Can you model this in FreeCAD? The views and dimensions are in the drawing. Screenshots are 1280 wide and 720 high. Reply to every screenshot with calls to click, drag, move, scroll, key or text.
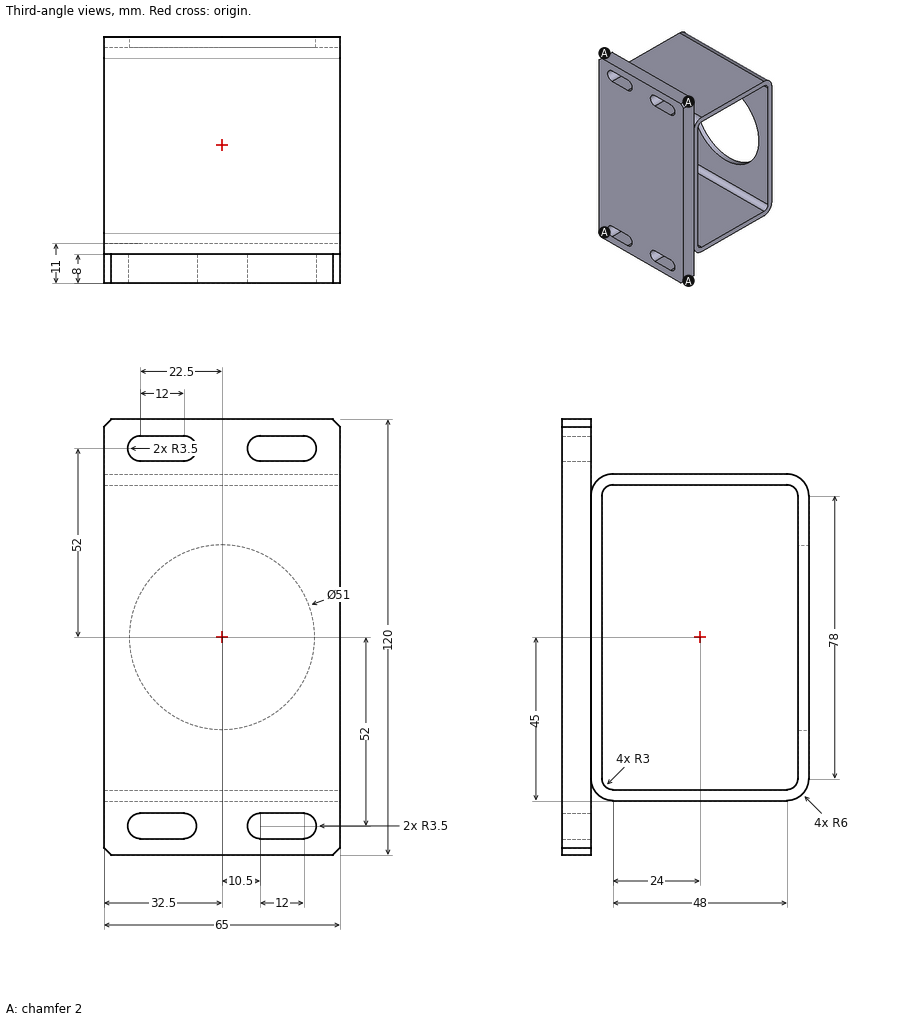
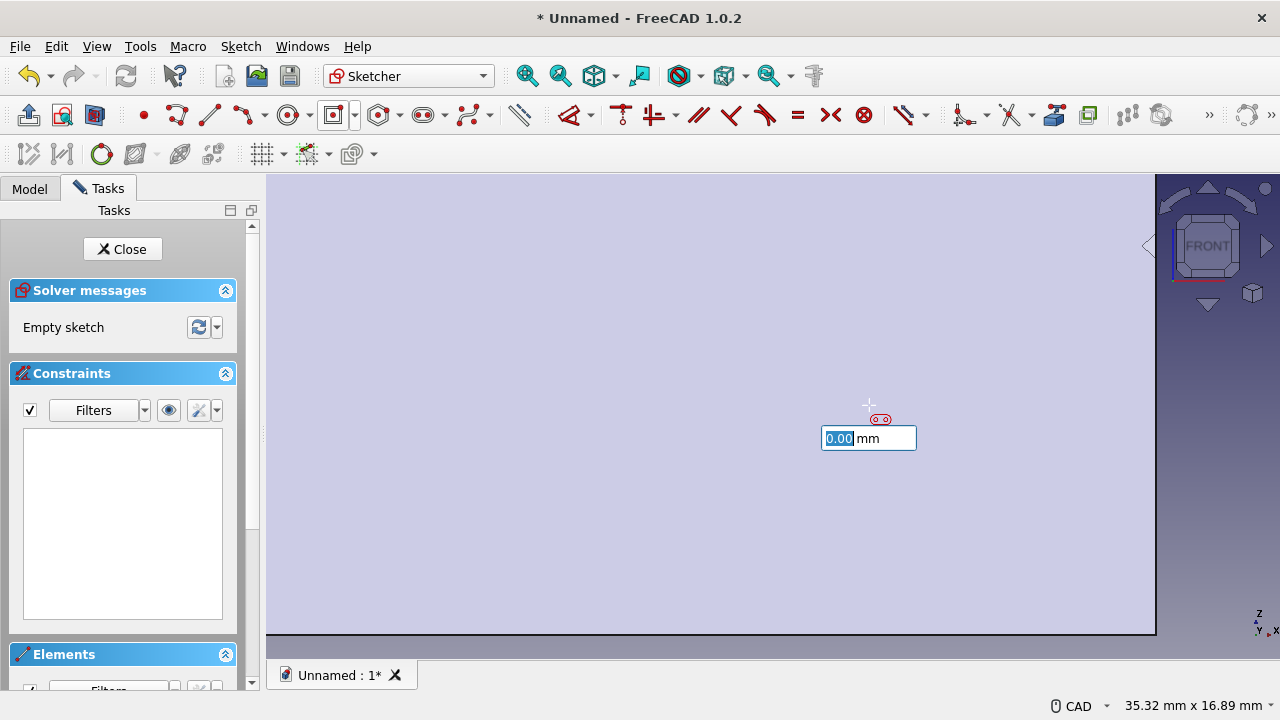
click(696, 506)
key(Escape)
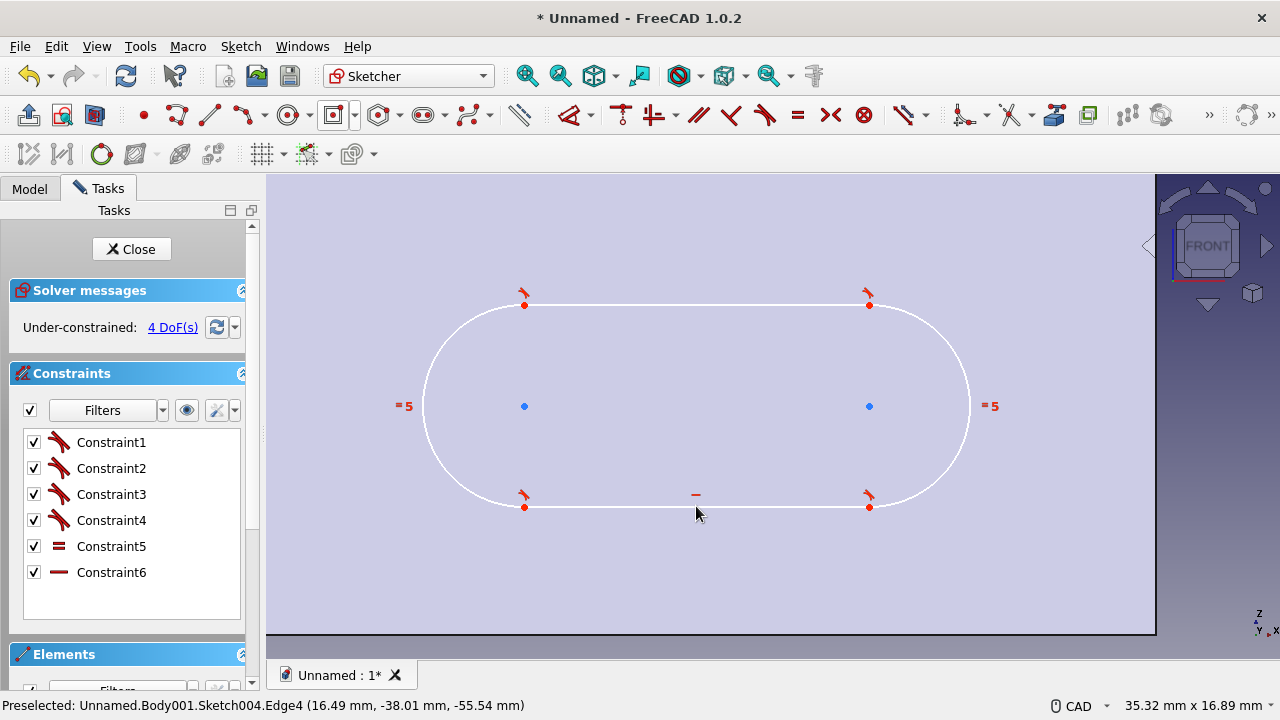
click(568, 116)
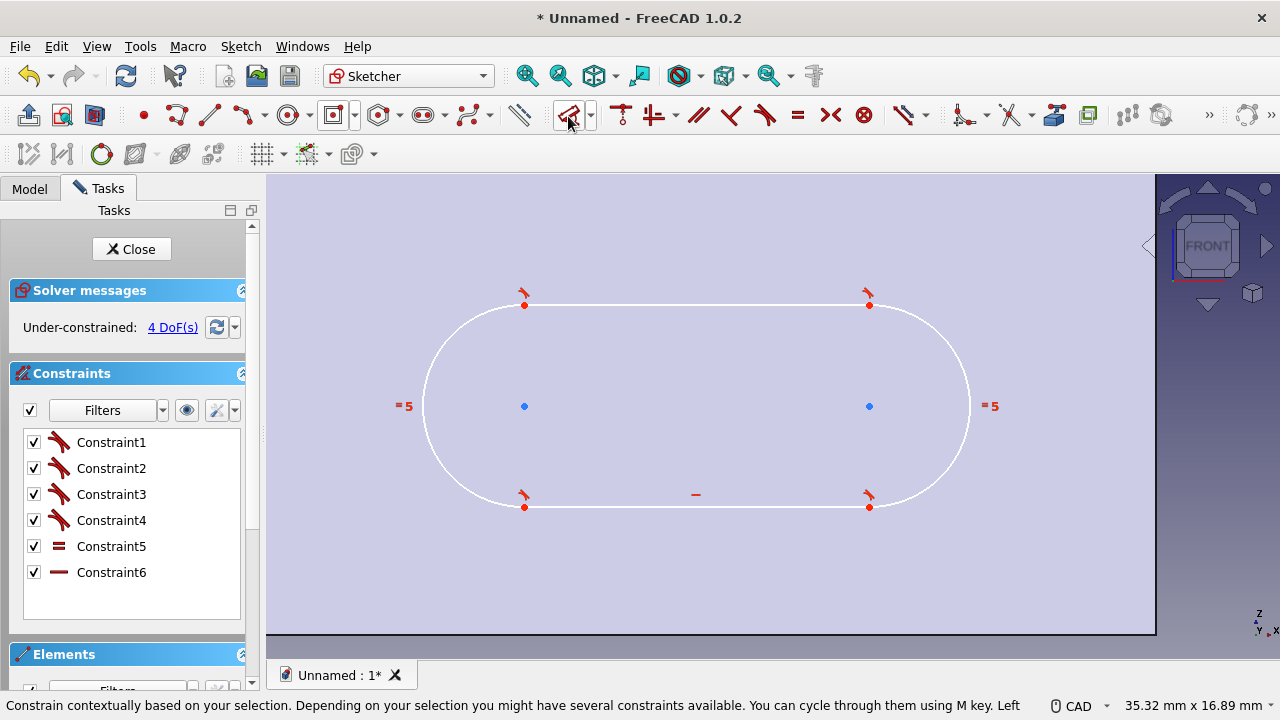
click(442, 347)
click(416, 328)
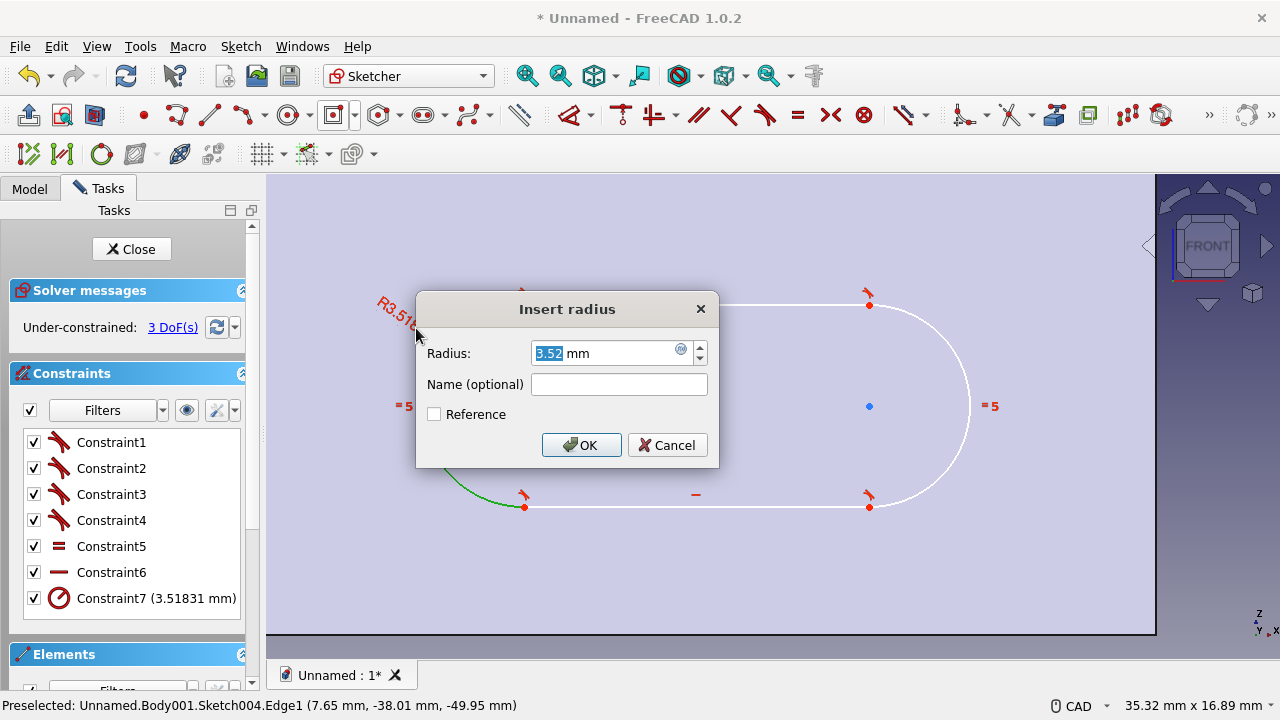
text(3.5)
key(Return)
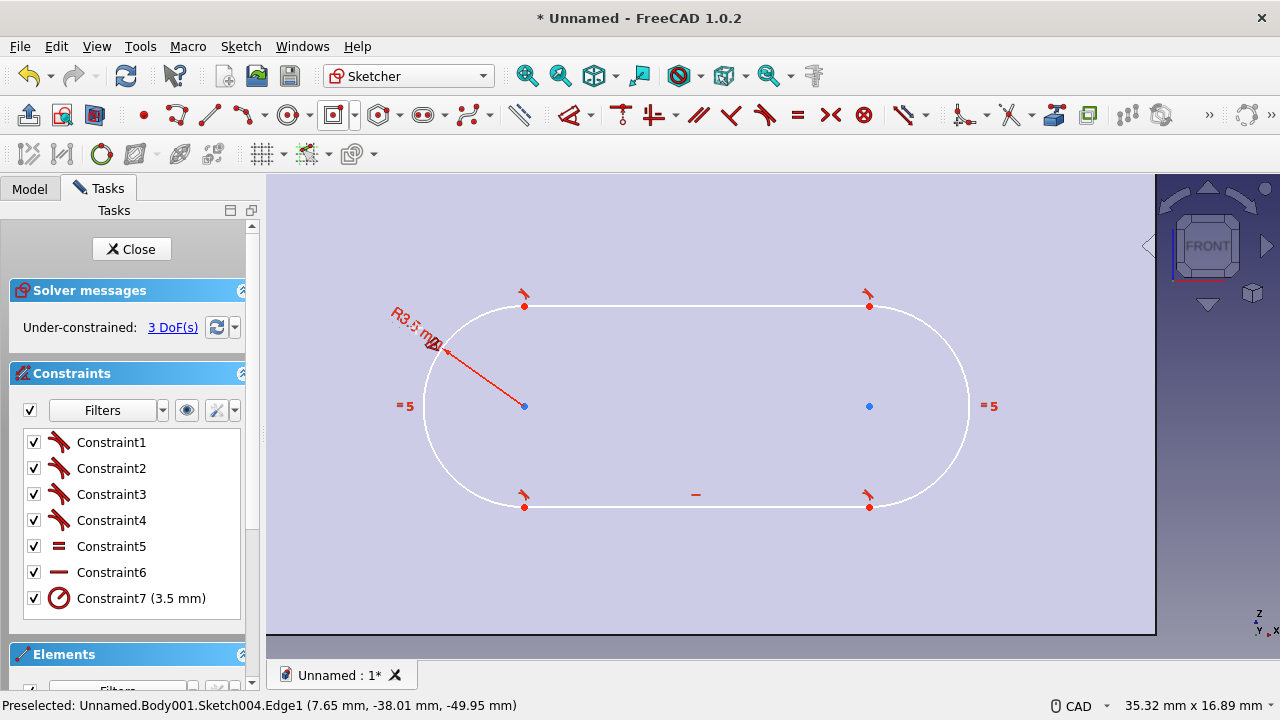
click(627, 306)
click(696, 272)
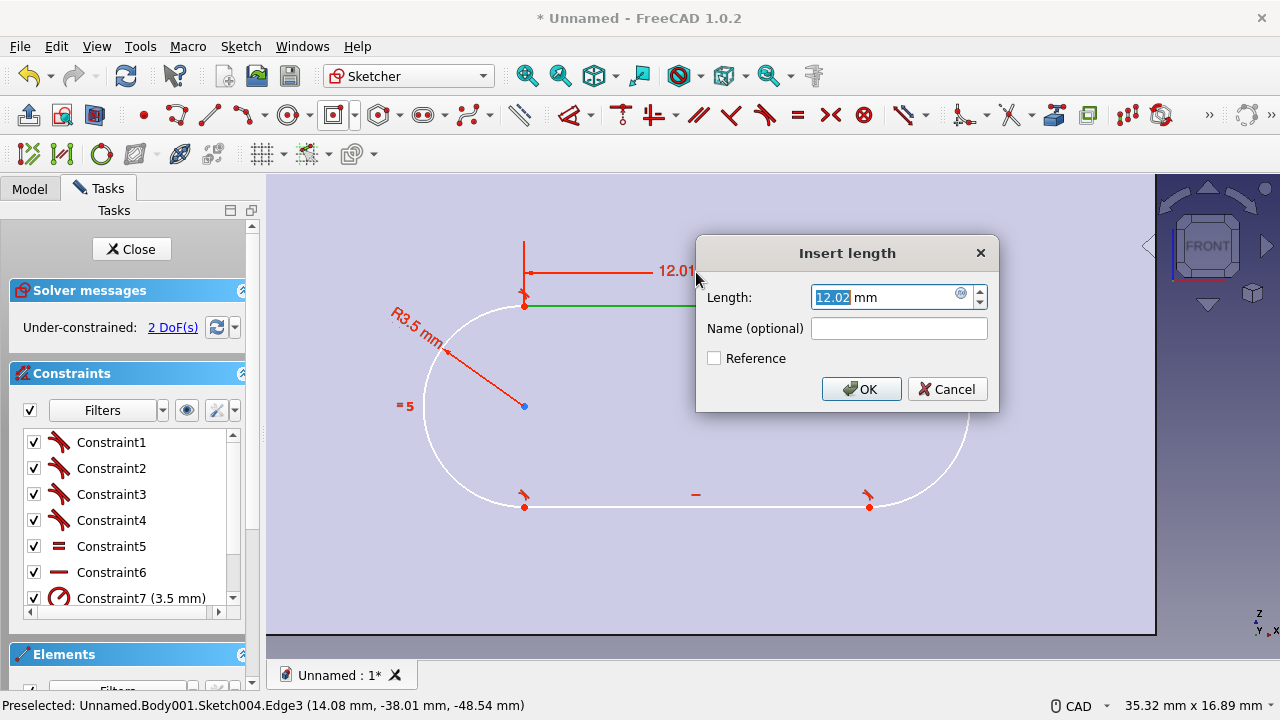
text(12)
key(Return)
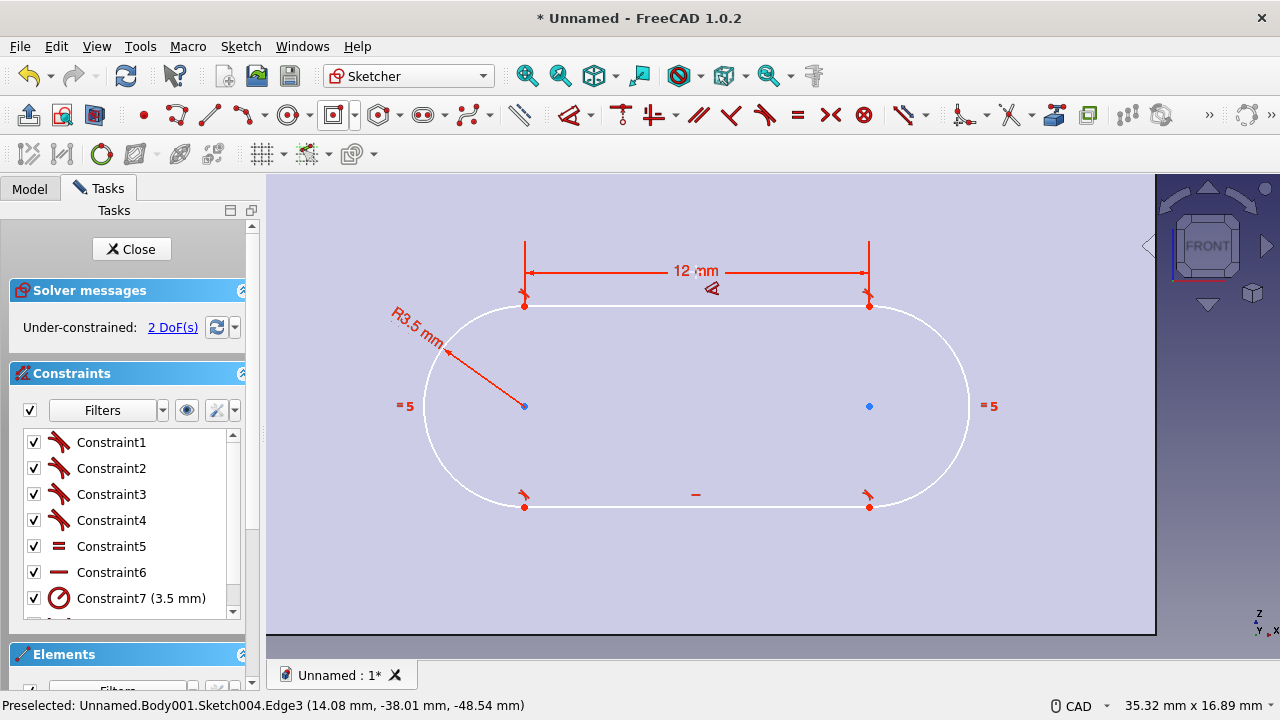
click(525, 407)
click(559, 257)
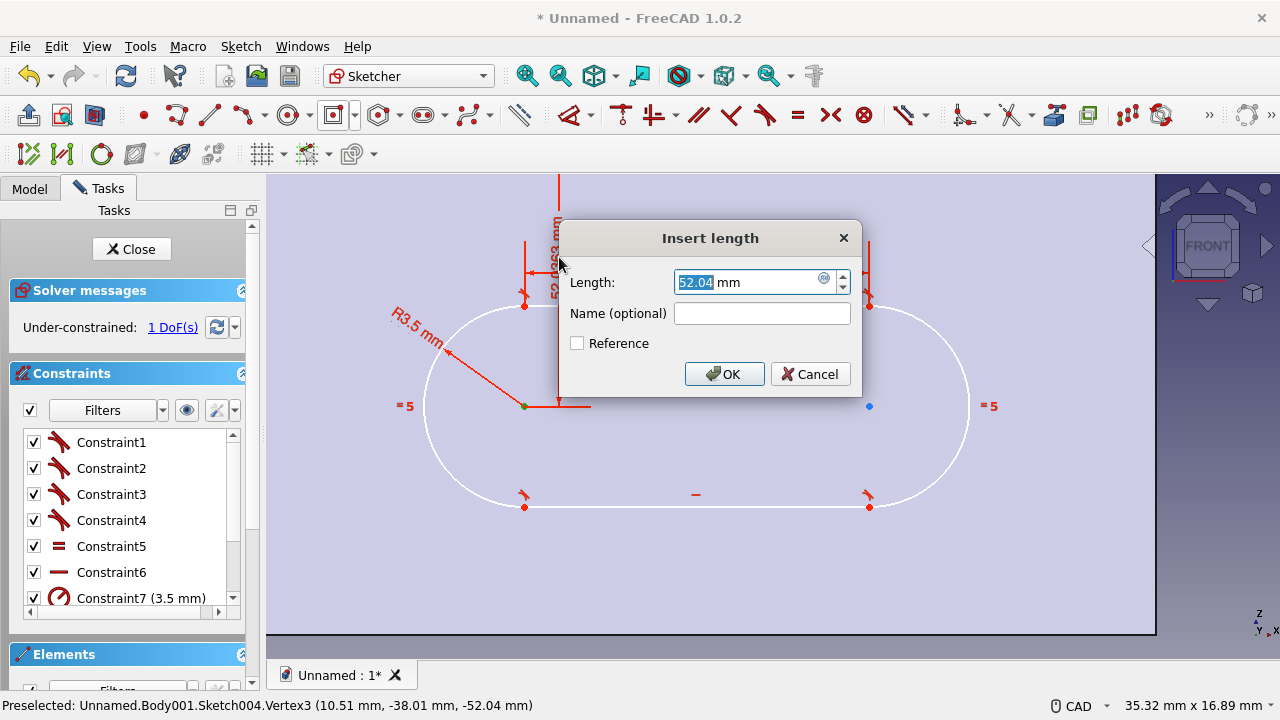
text(52)
key(Return)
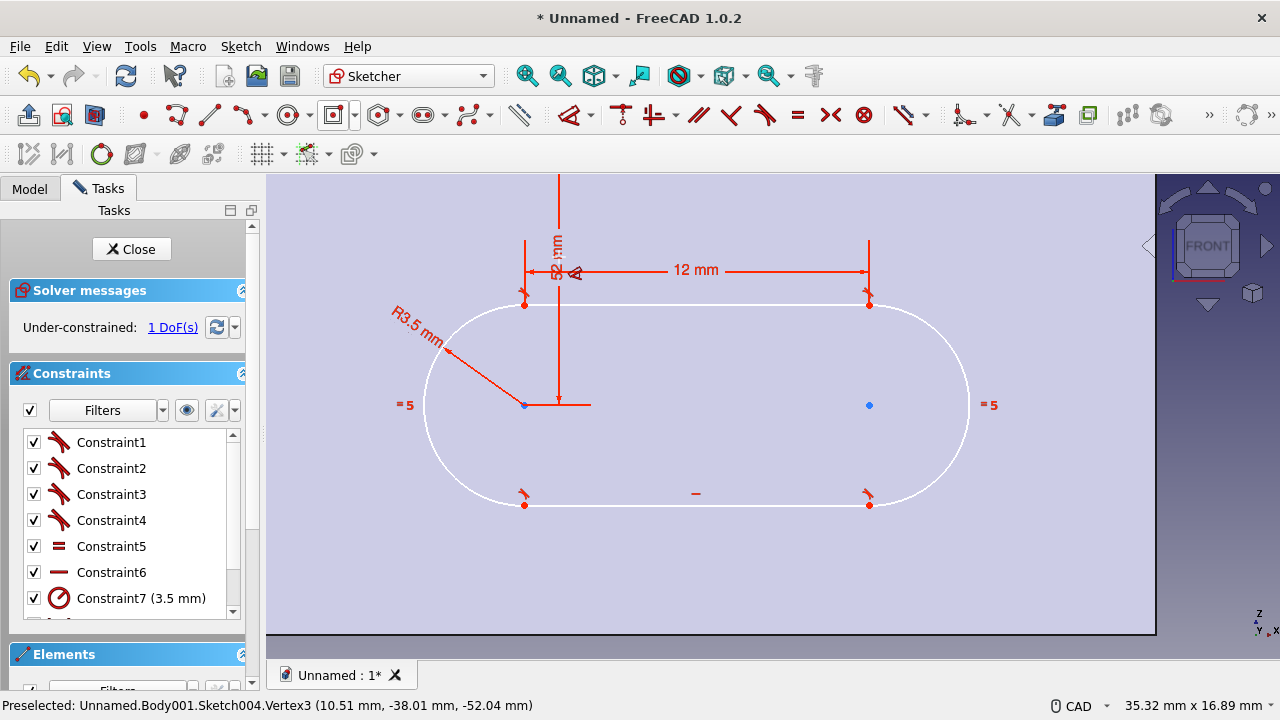
click(525, 305)
click(329, 339)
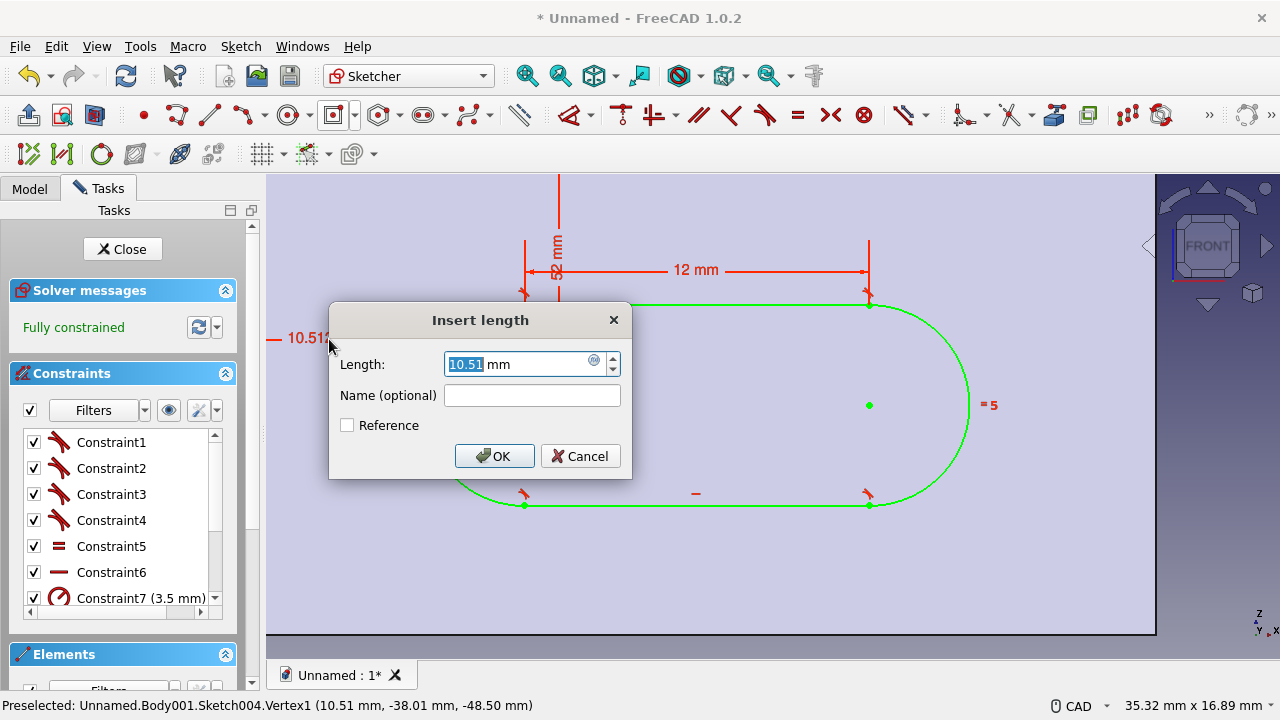
text(10.5)
key(Return)
key(Escape)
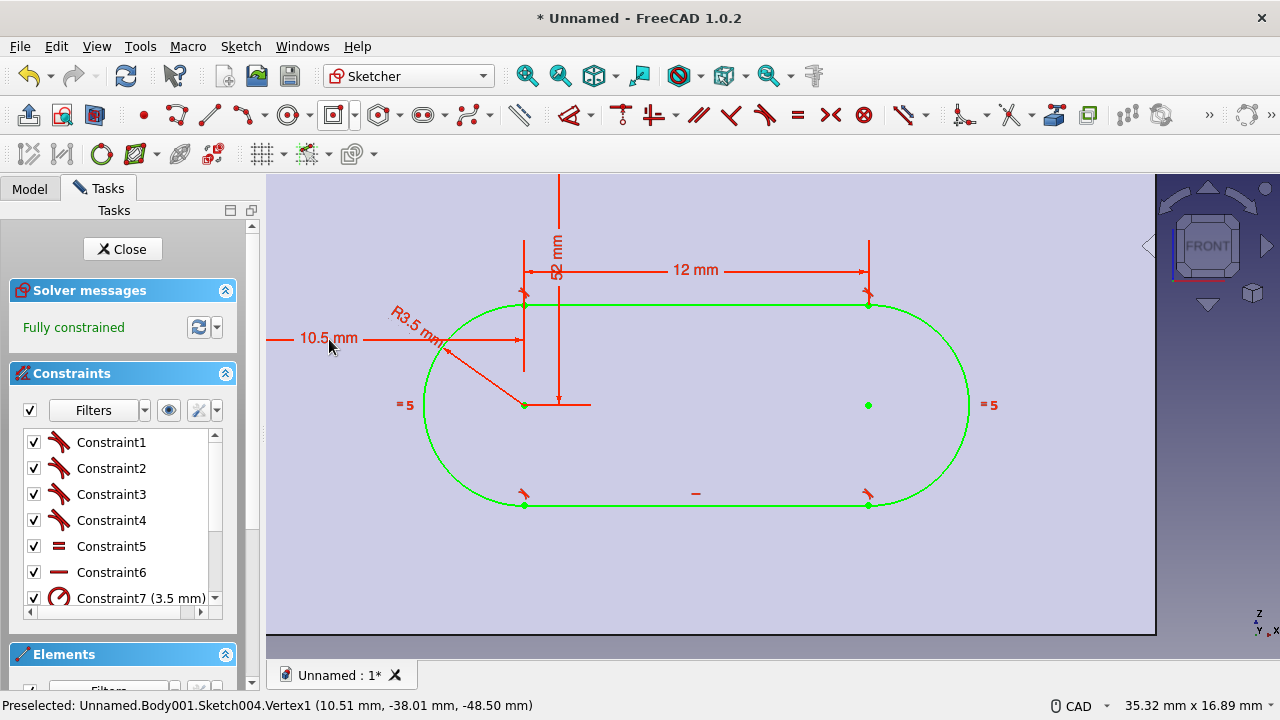
click(123, 249)